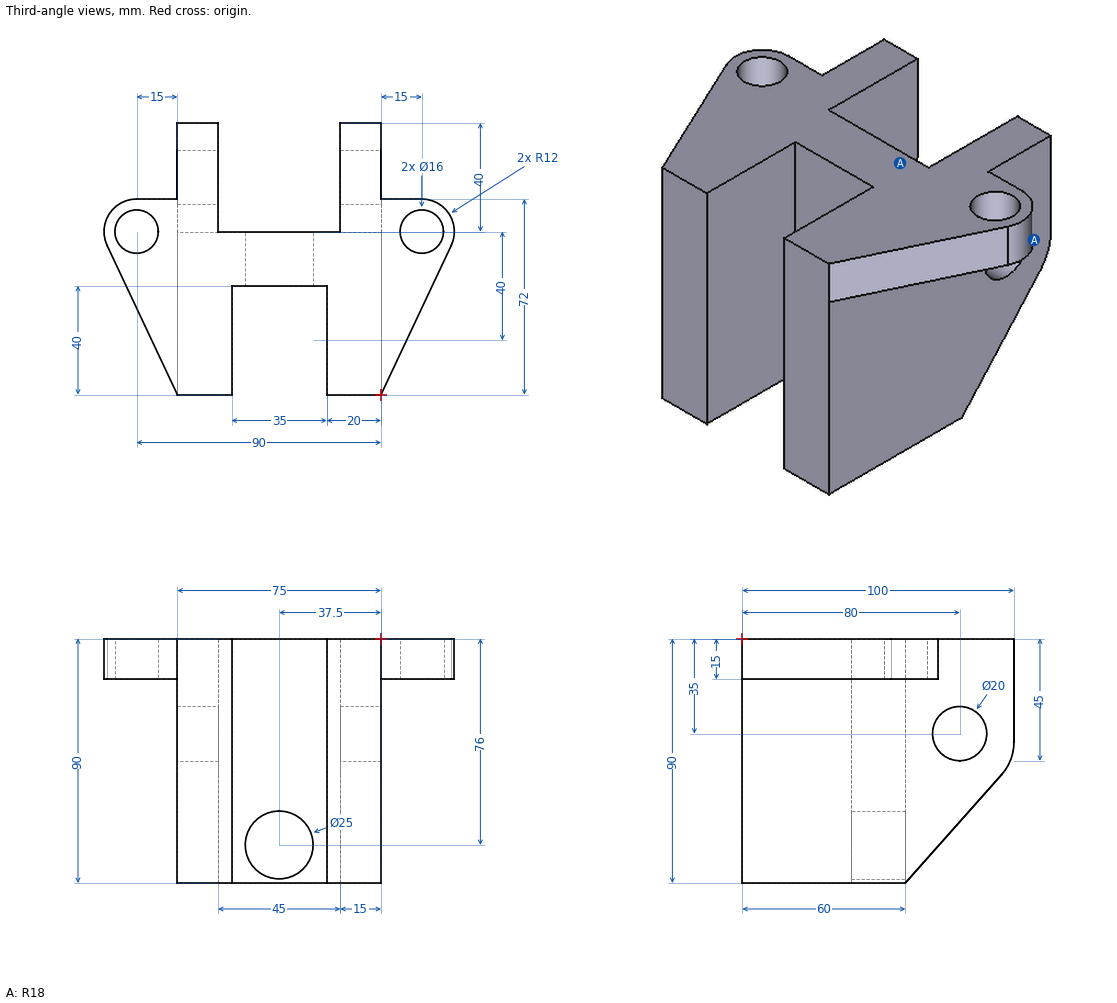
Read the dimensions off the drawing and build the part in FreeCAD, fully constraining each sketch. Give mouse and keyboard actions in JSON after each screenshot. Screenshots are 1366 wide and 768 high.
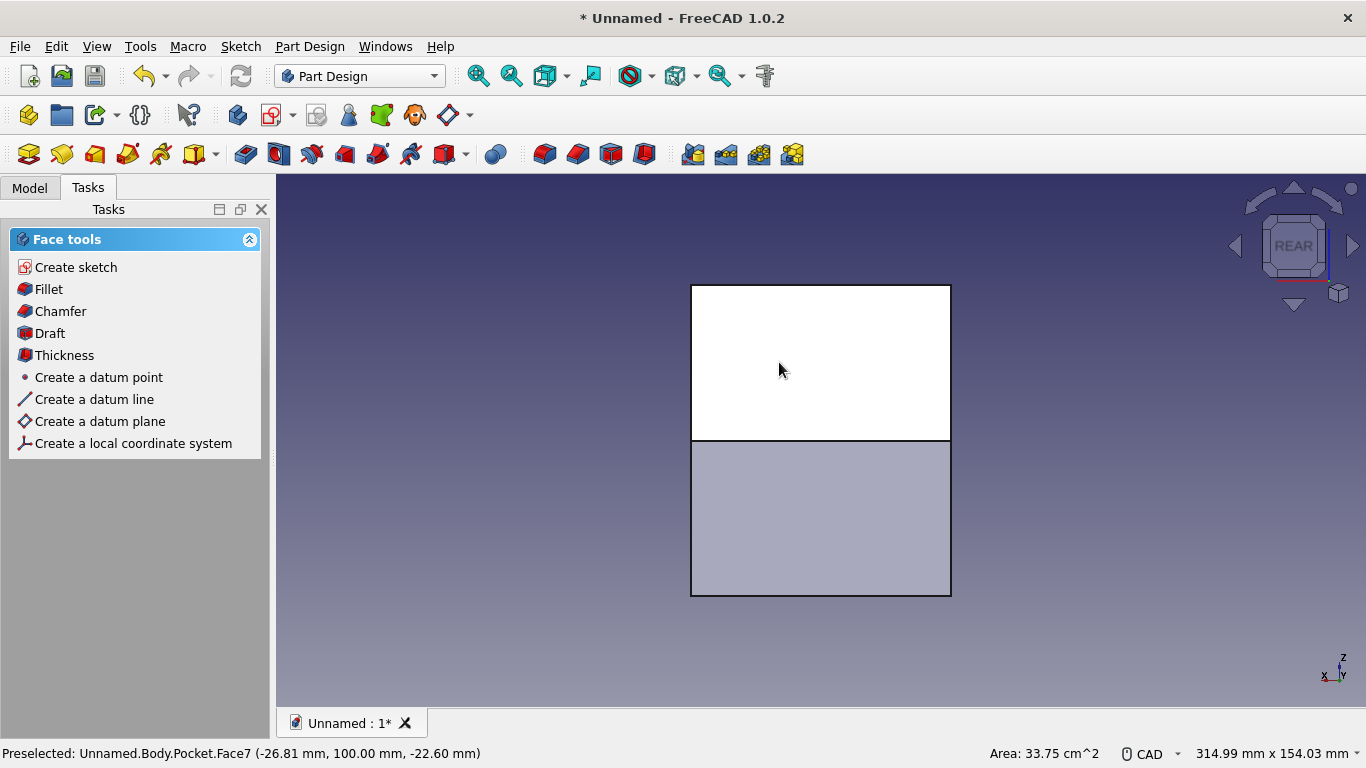
{"action": "left_click", "coordinate": [270, 116]}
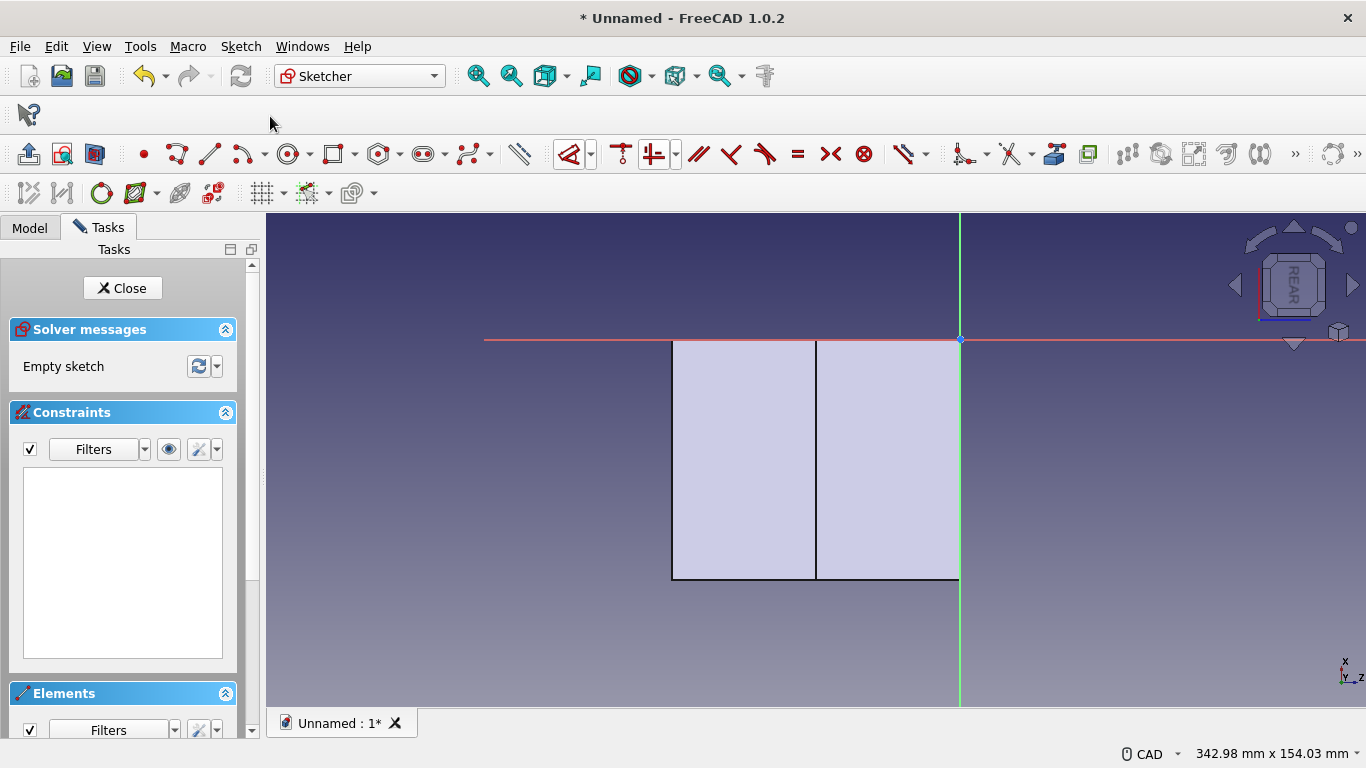
{"action": "scroll", "coordinate": [955, 387], "scroll_direction": "up", "scroll_amount": 2}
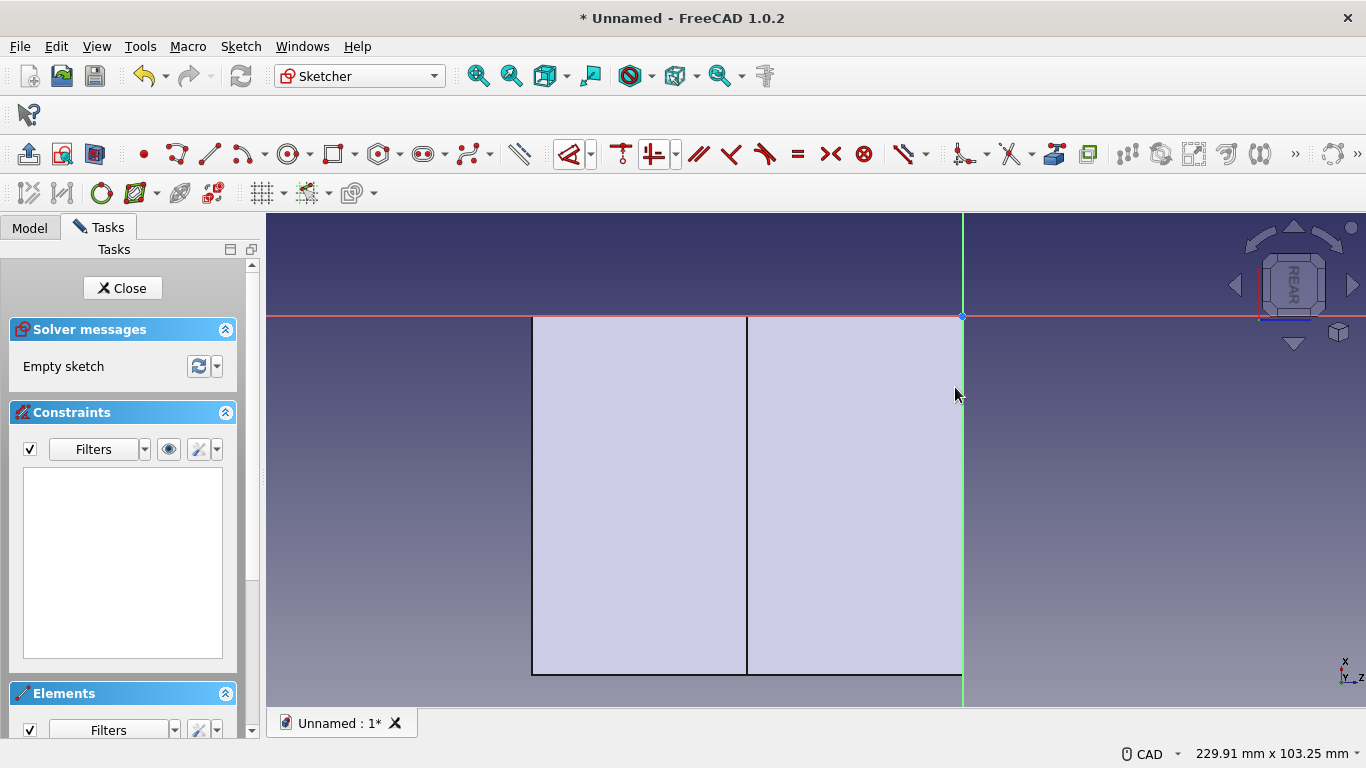
{"action": "key", "text": "g r"}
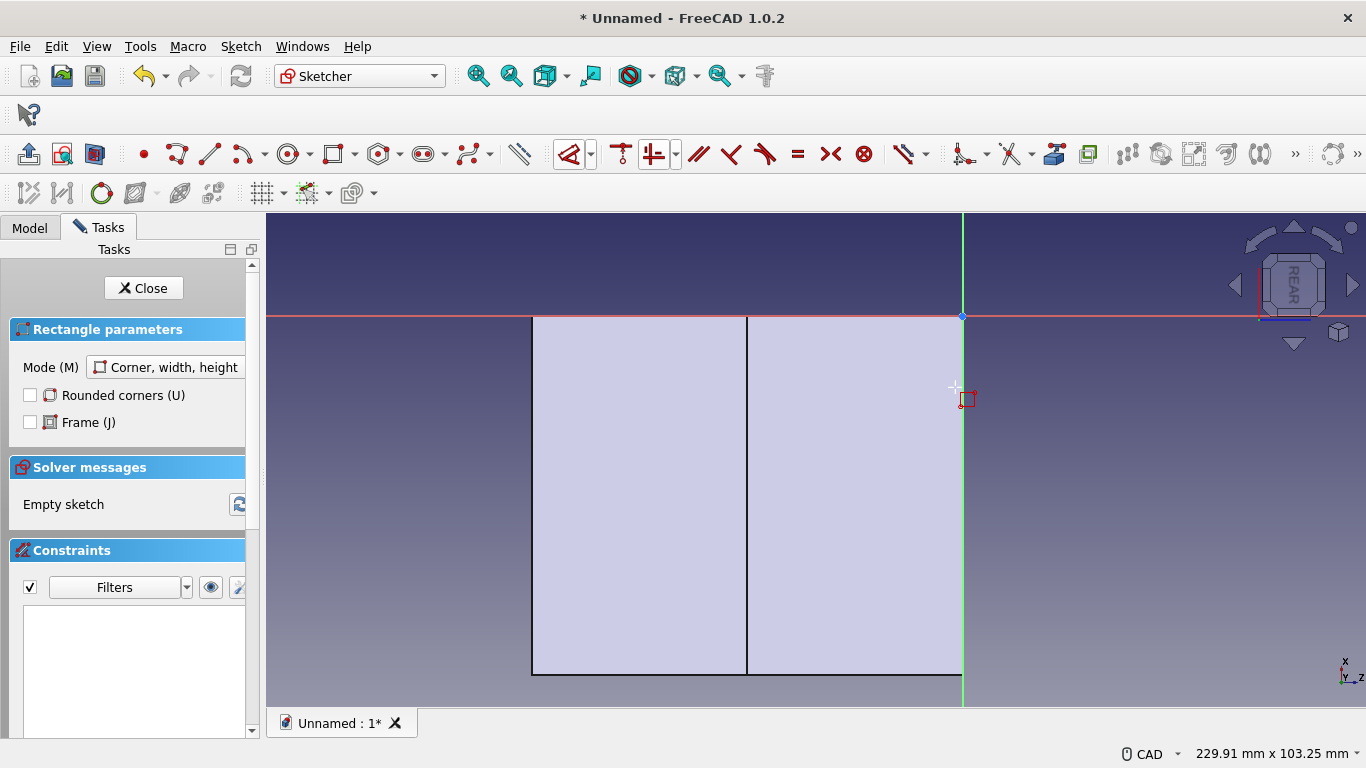
{"action": "left_click", "coordinate": [532, 388]}
{"action": "left_click", "coordinate": [963, 603]}
{"action": "key", "text": "Escape"}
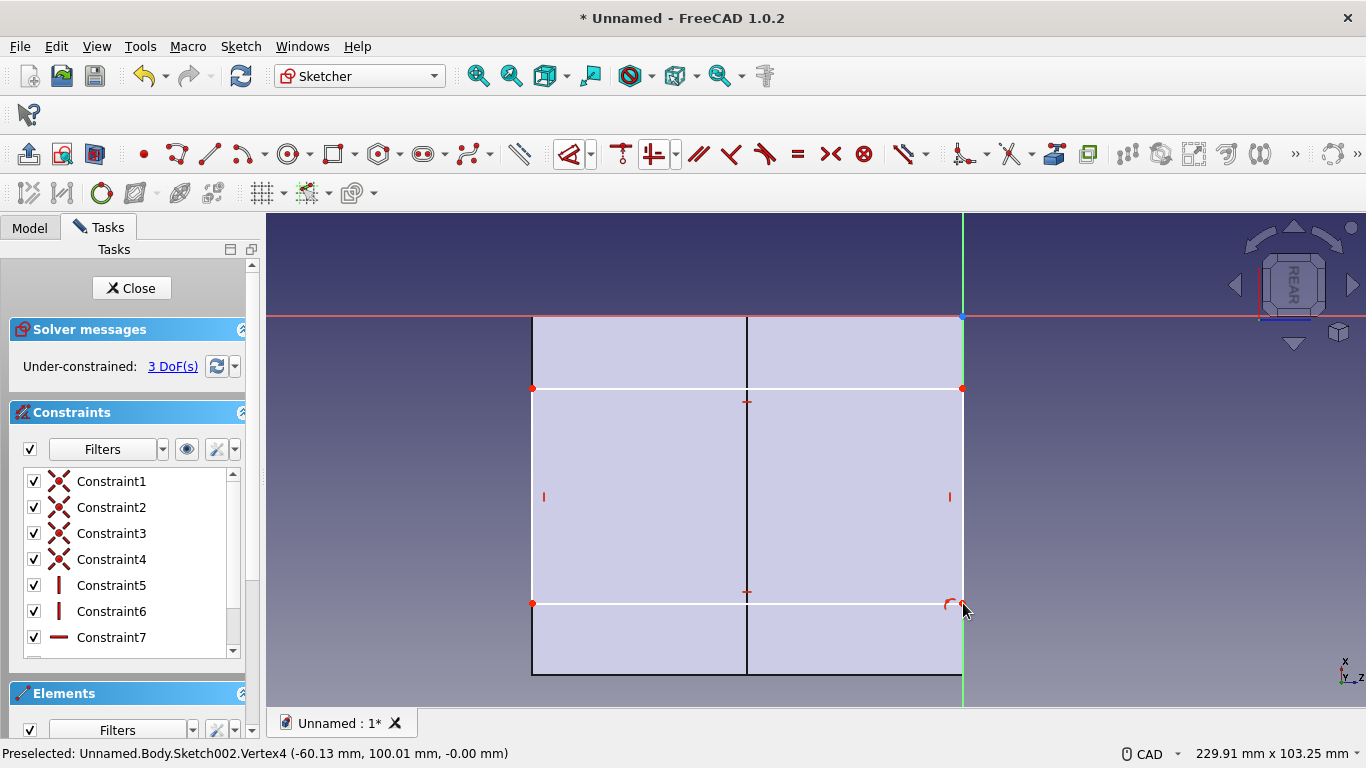
{"action": "left_click", "coordinate": [532, 454]}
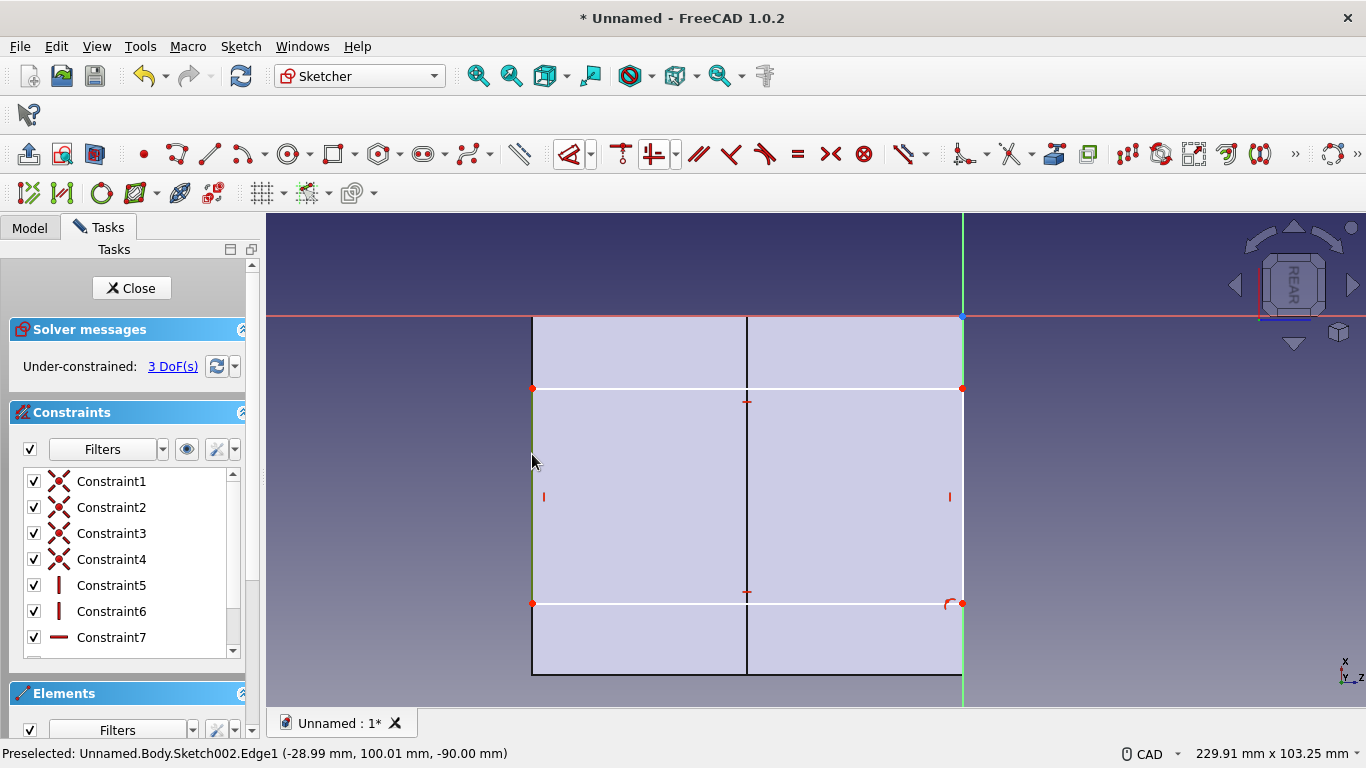
{"action": "left_click", "coordinate": [590, 154]}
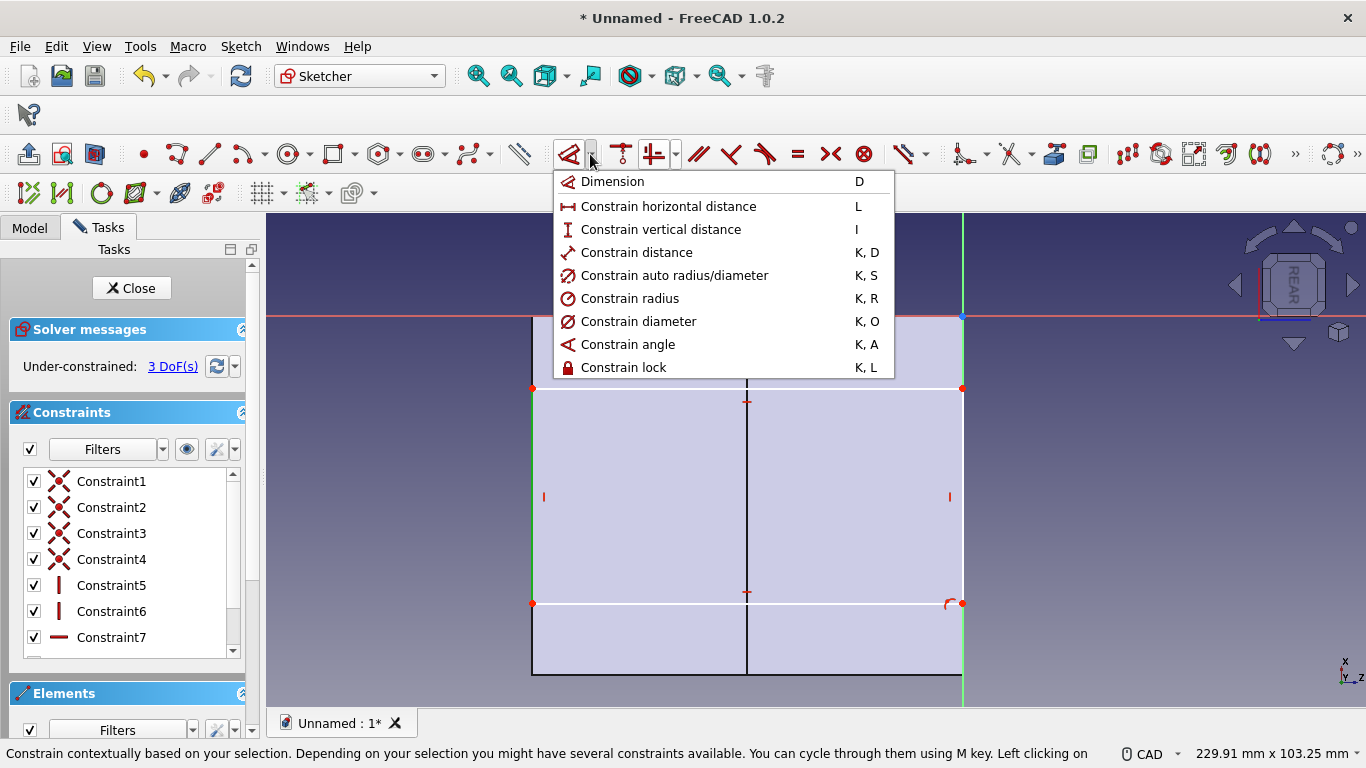
{"action": "left_click", "coordinate": [724, 230]}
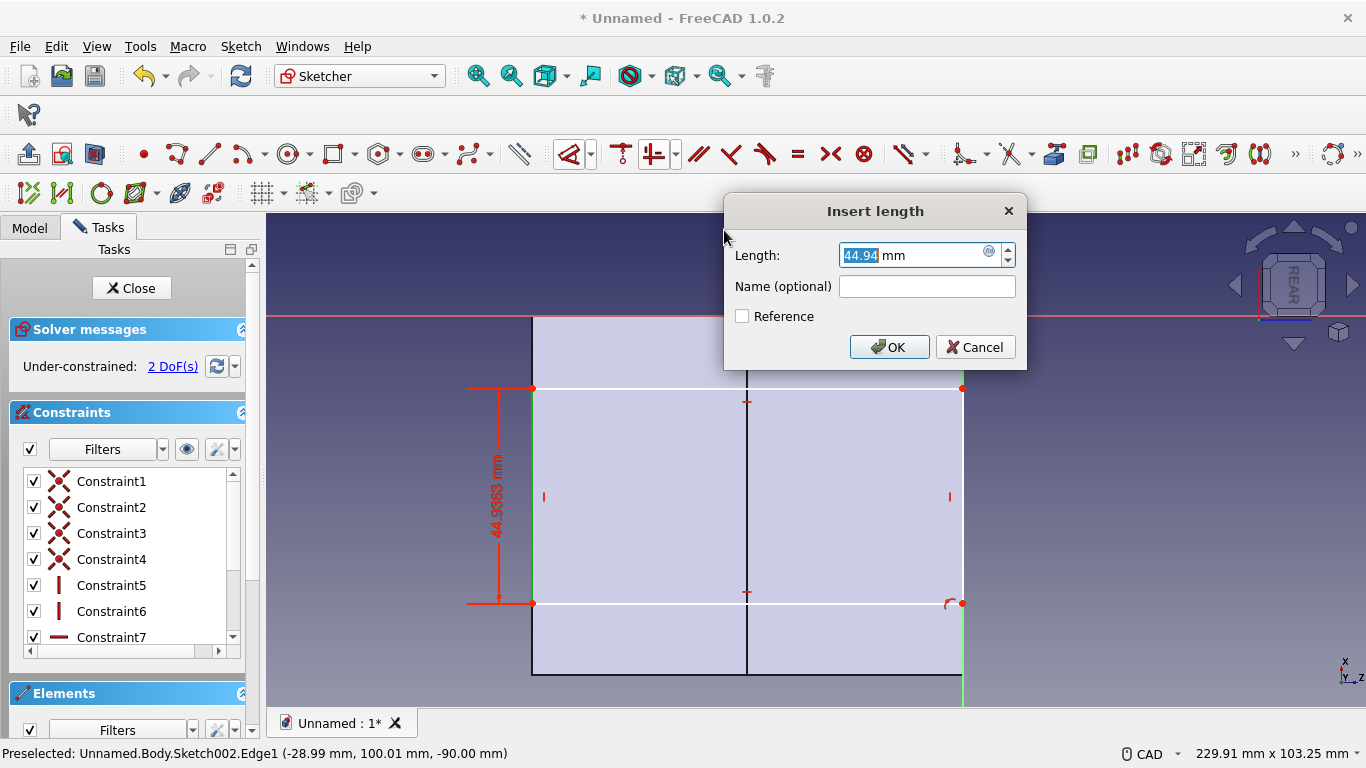
{"action": "type", "text": "45"}
{"action": "key", "text": "Return"}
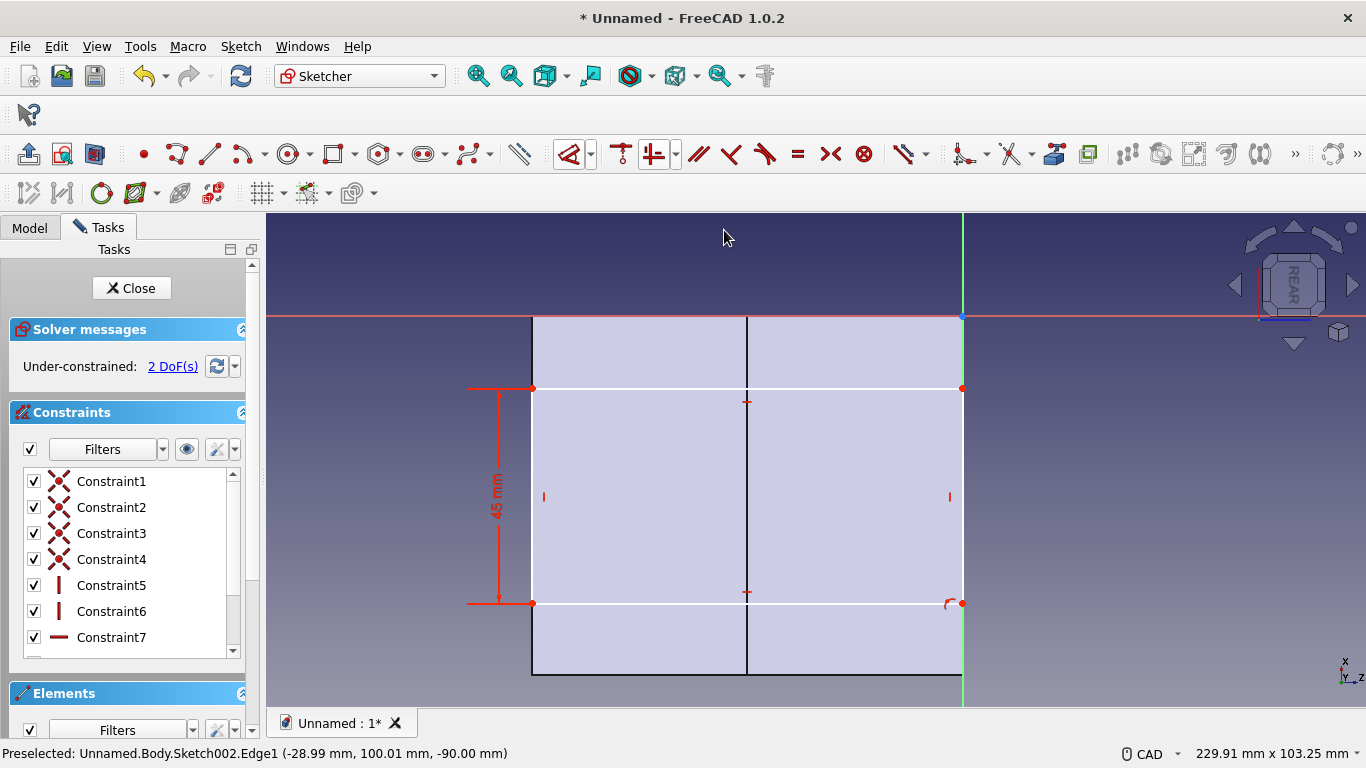
{"action": "left_click", "coordinate": [661, 604]}